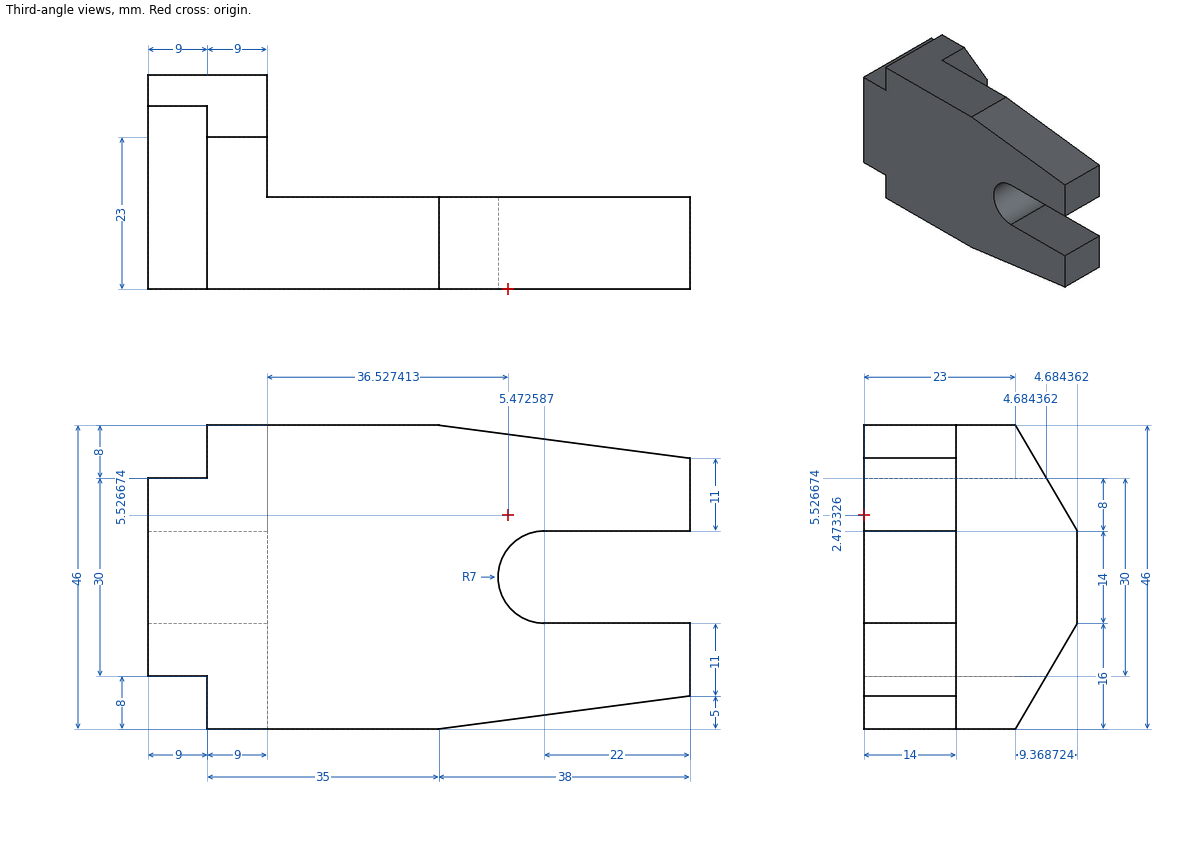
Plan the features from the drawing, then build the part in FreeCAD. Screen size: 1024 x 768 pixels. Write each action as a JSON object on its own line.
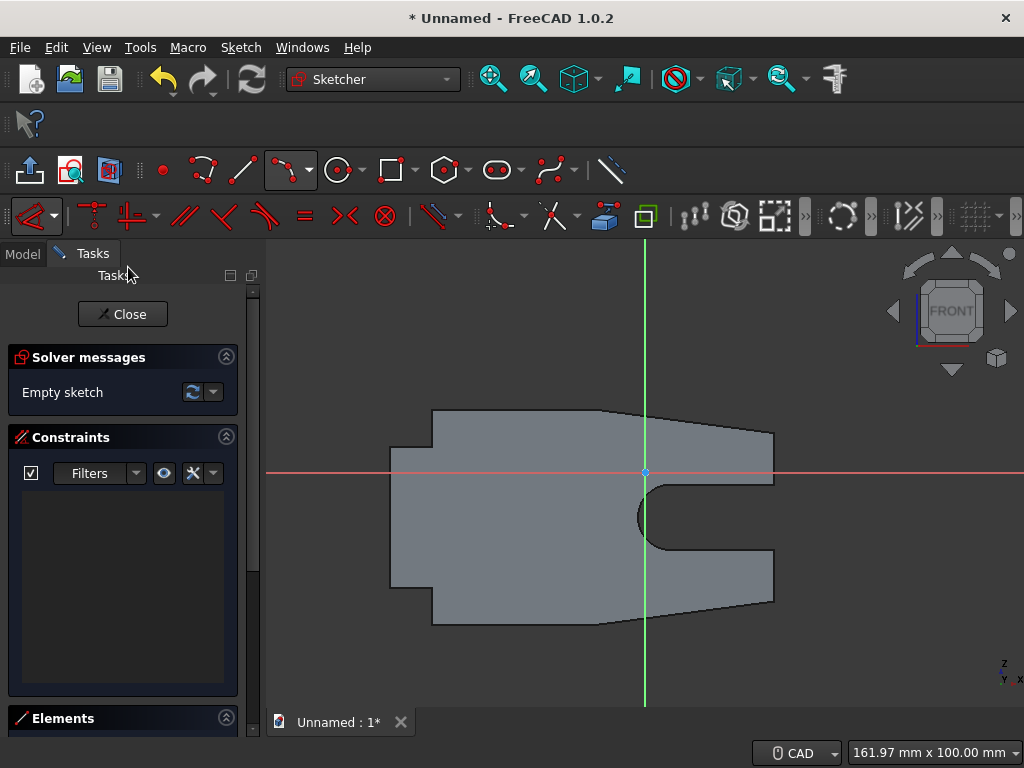
{"action": "scroll", "coordinate": [397, 607], "scroll_direction": "up", "scroll_amount": 2}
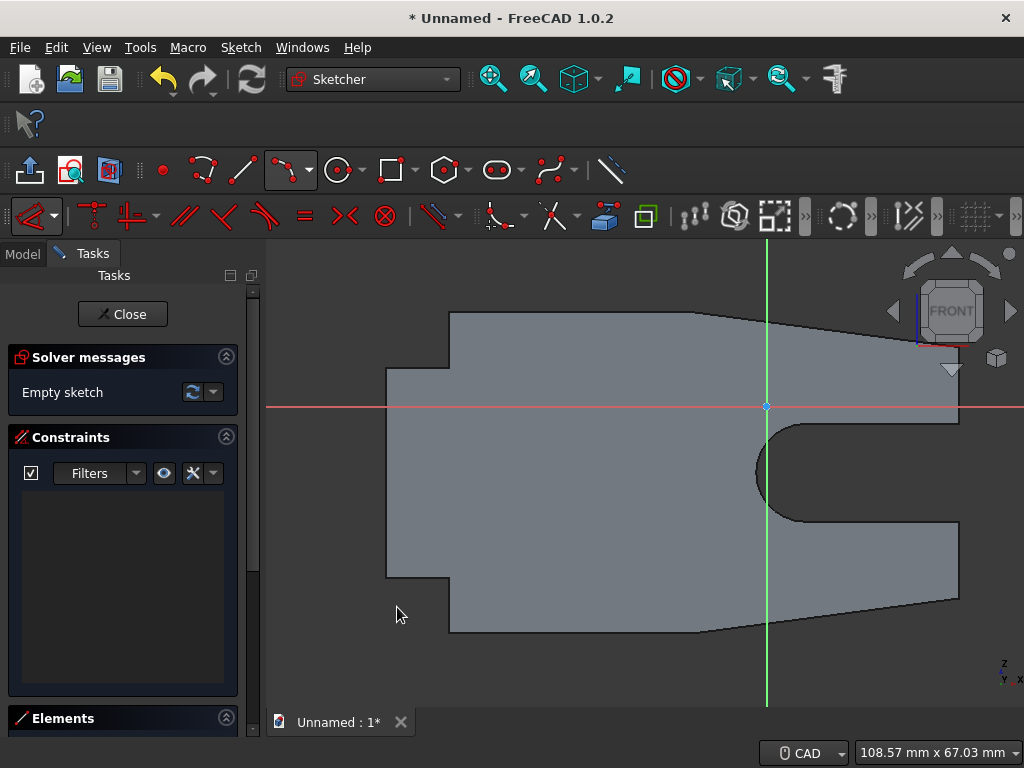
{"action": "left_click", "coordinate": [204, 170]}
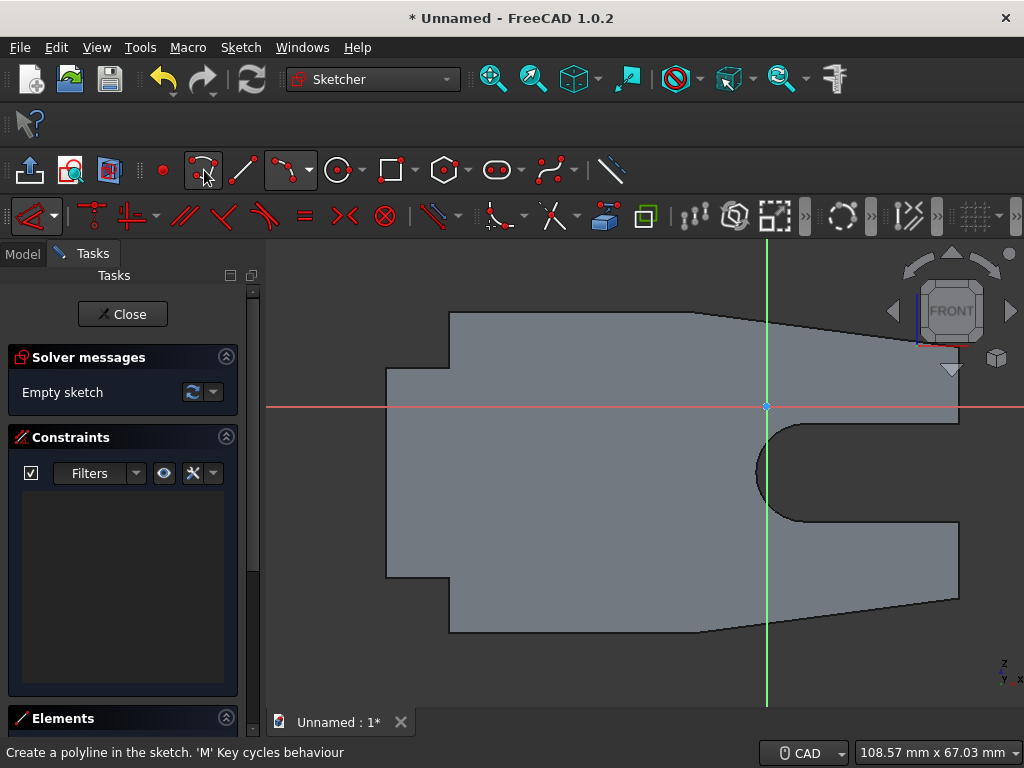
{"action": "left_click", "coordinate": [512, 312]}
{"action": "left_click", "coordinate": [512, 633]}
{"action": "left_click", "coordinate": [449, 633]}
{"action": "left_click", "coordinate": [449, 578]}
{"action": "left_click", "coordinate": [386, 578]}
{"action": "left_click", "coordinate": [386, 368]}
{"action": "left_click", "coordinate": [449, 368]}
{"action": "left_click", "coordinate": [449, 312]}
{"action": "left_click", "coordinate": [512, 313]}
{"action": "key", "text": "Escape"}
{"action": "key", "text": "Escape"}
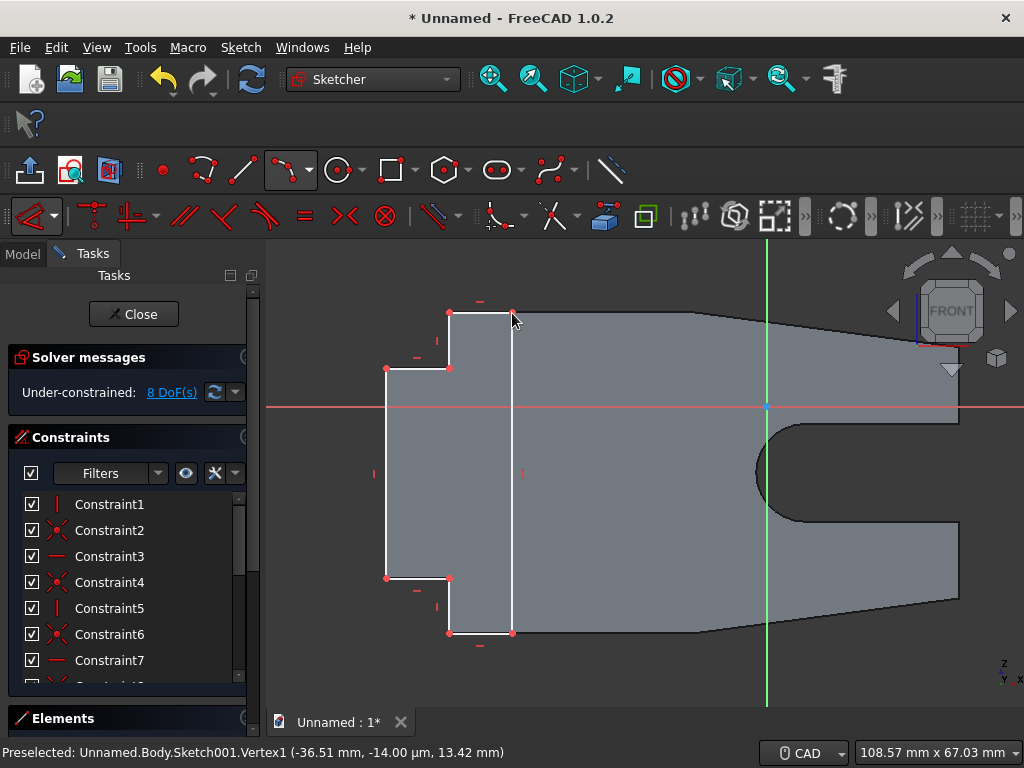
{"action": "left_click", "coordinate": [493, 634]}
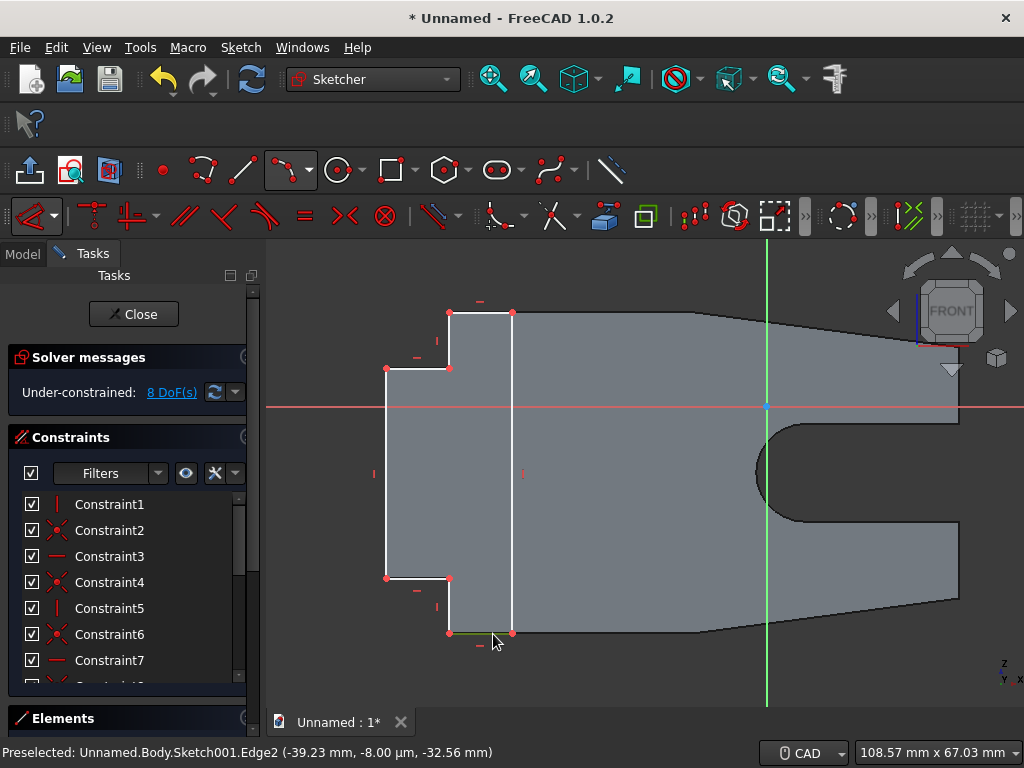
{"action": "key", "text": "l"}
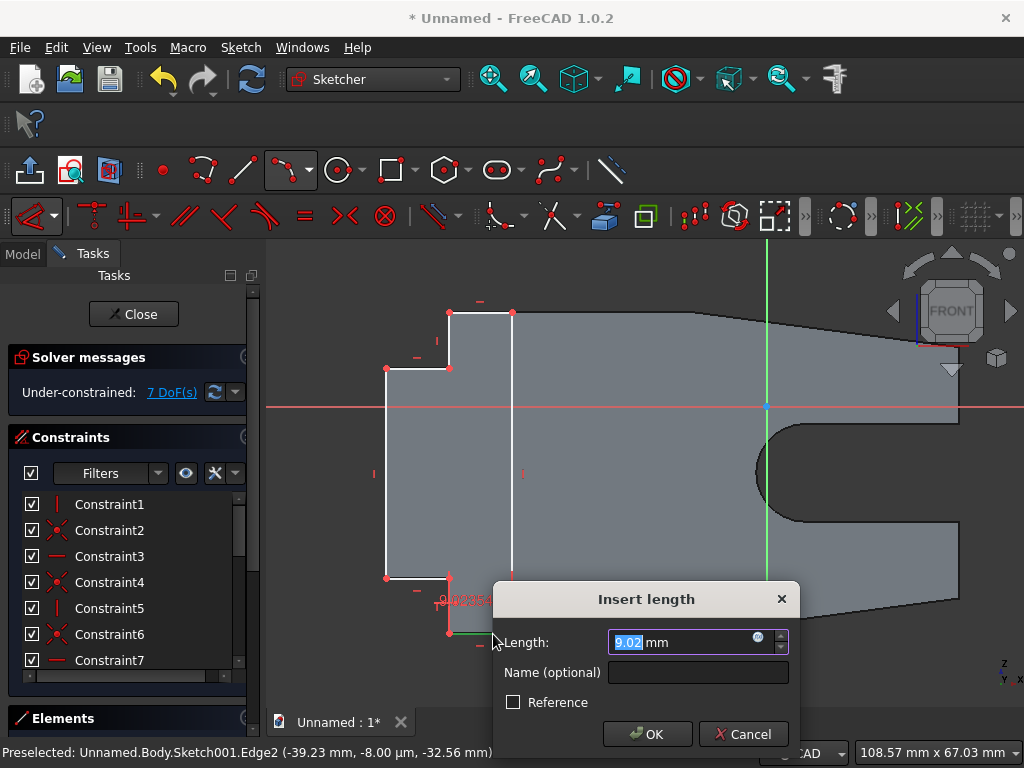
{"action": "type", "text": "9"}
{"action": "key", "text": "Return"}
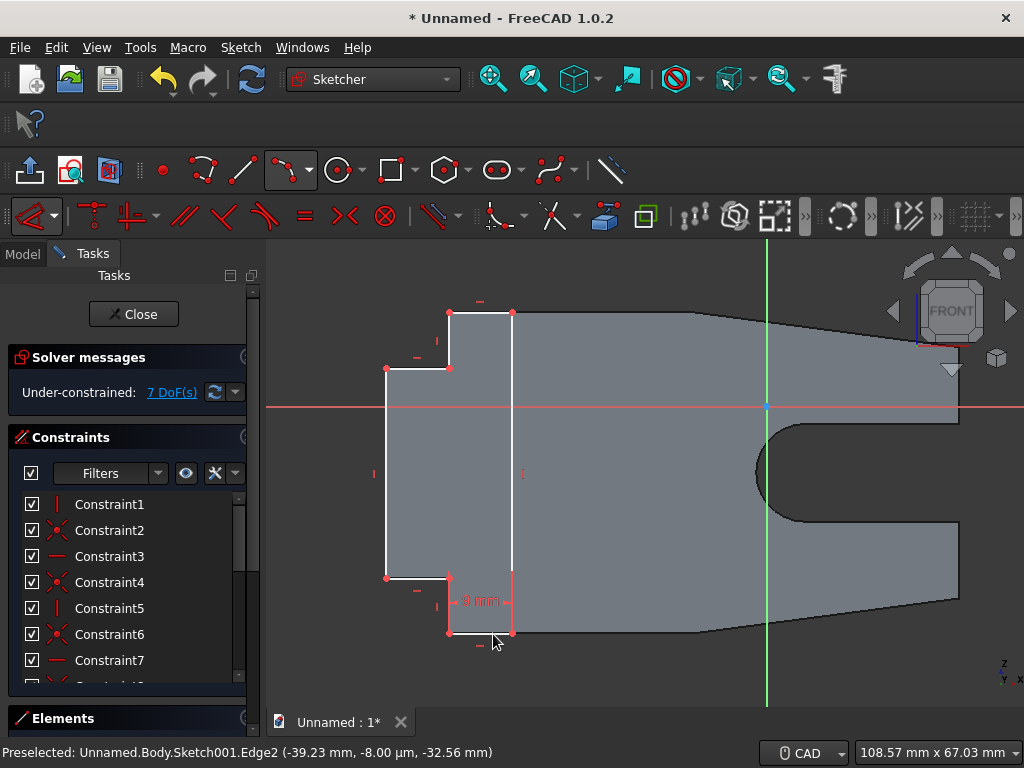
{"action": "left_click", "coordinate": [449, 617]}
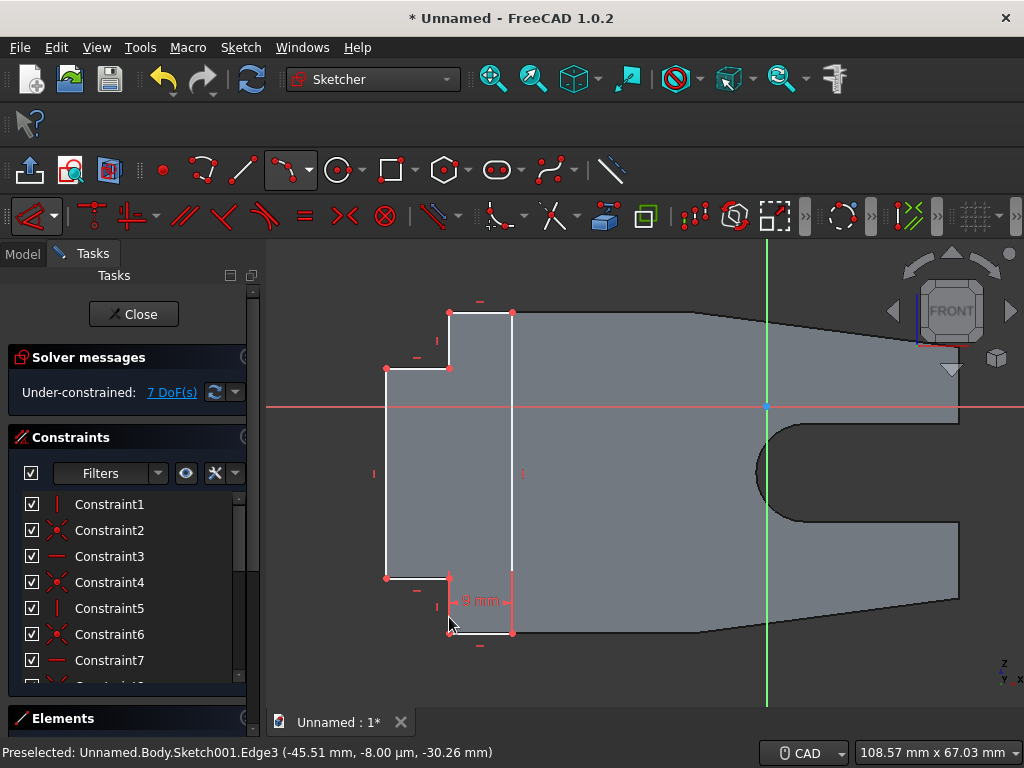
{"action": "left_click", "coordinate": [56, 216]}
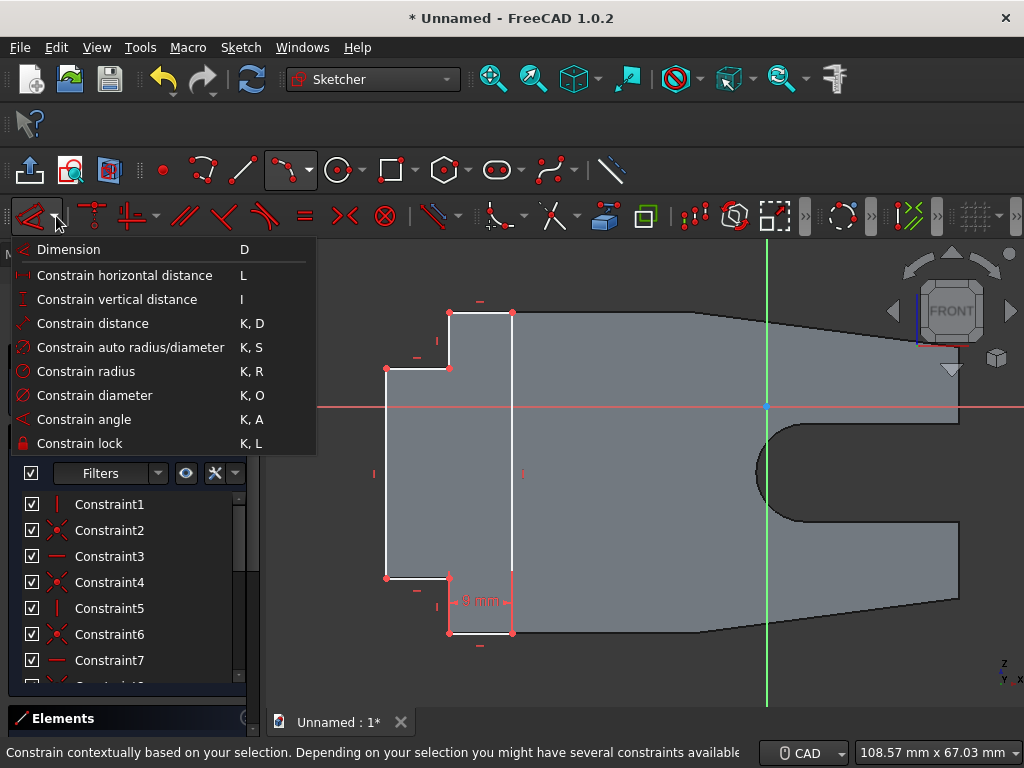
{"action": "left_click", "coordinate": [164, 299]}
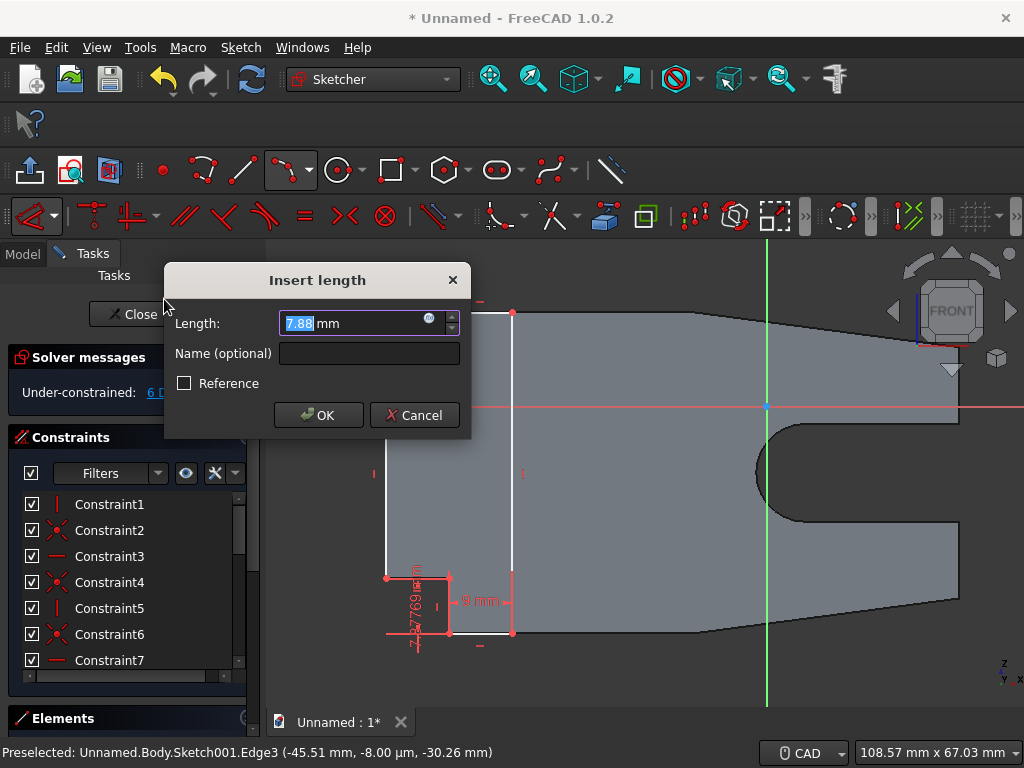
{"action": "type", "text": "8"}
{"action": "key", "text": "Return"}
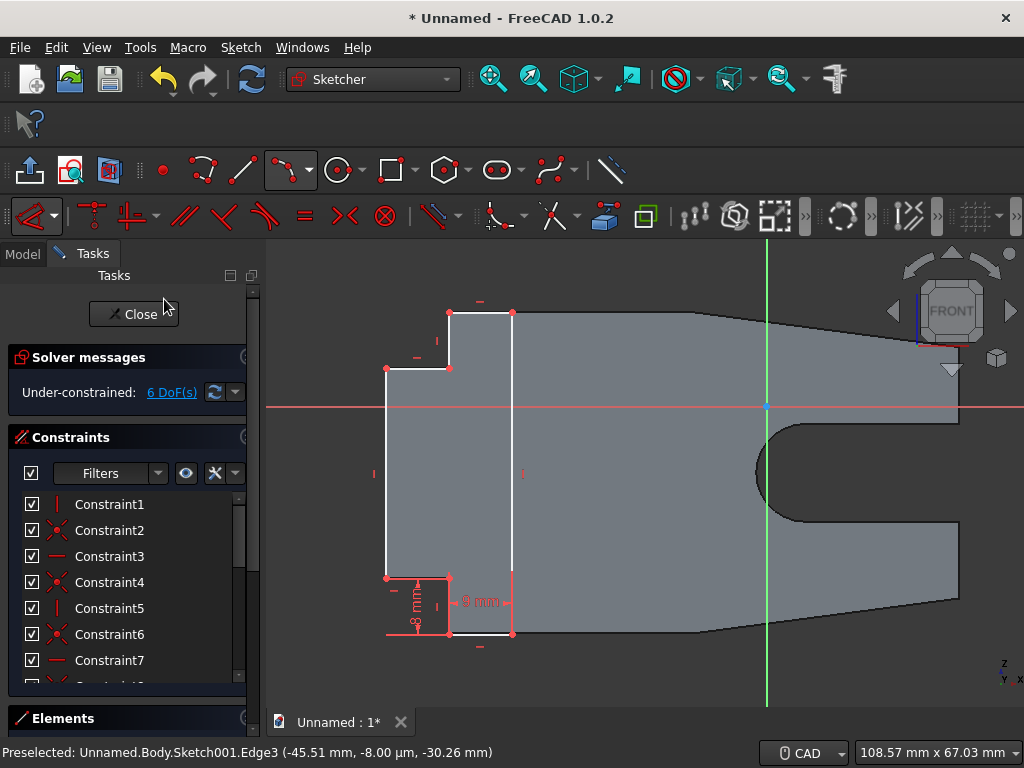
{"action": "left_click", "coordinate": [430, 579]}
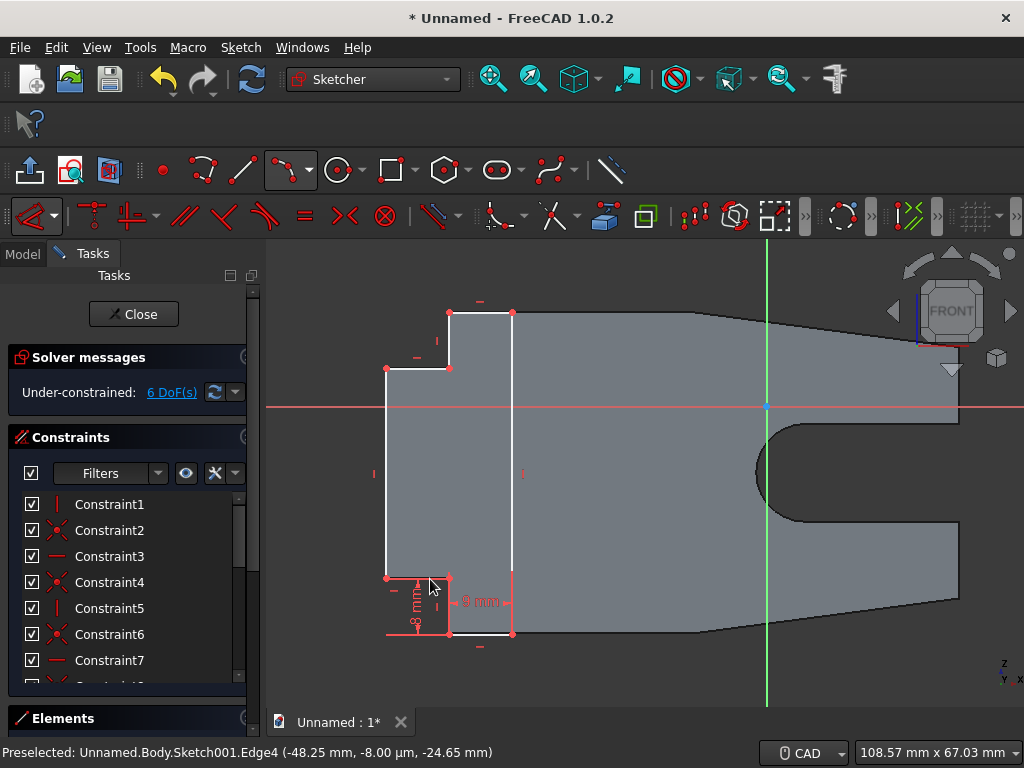
{"action": "left_click", "coordinate": [56, 216]}